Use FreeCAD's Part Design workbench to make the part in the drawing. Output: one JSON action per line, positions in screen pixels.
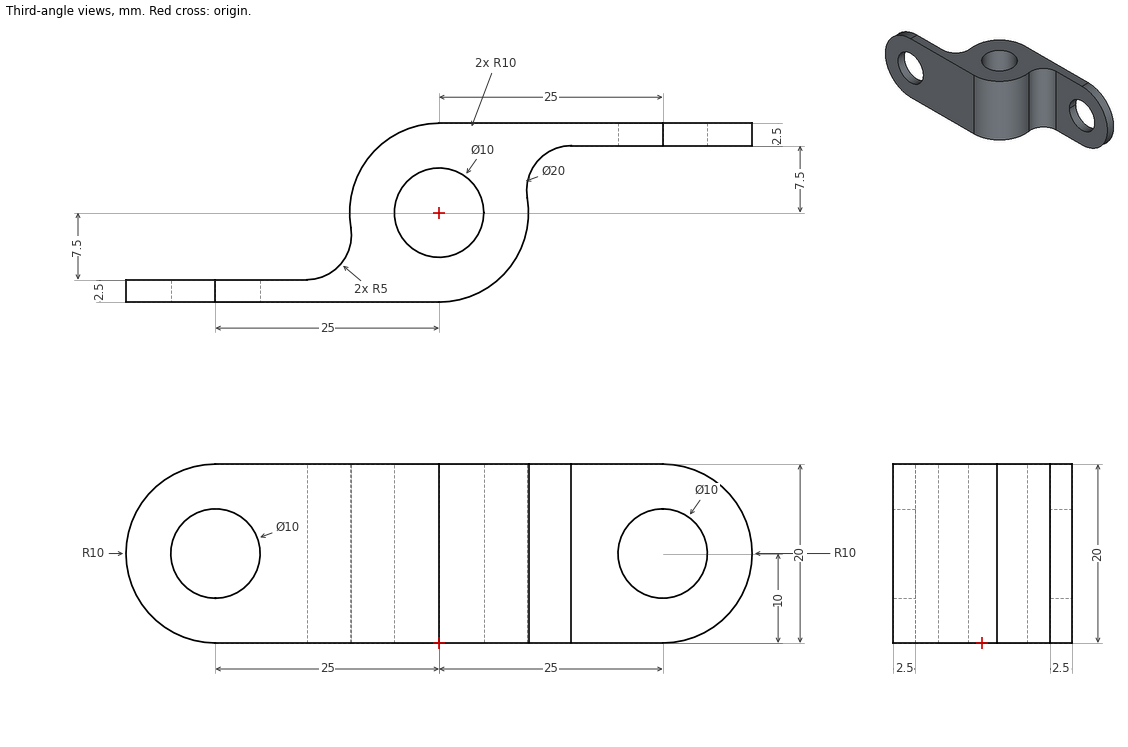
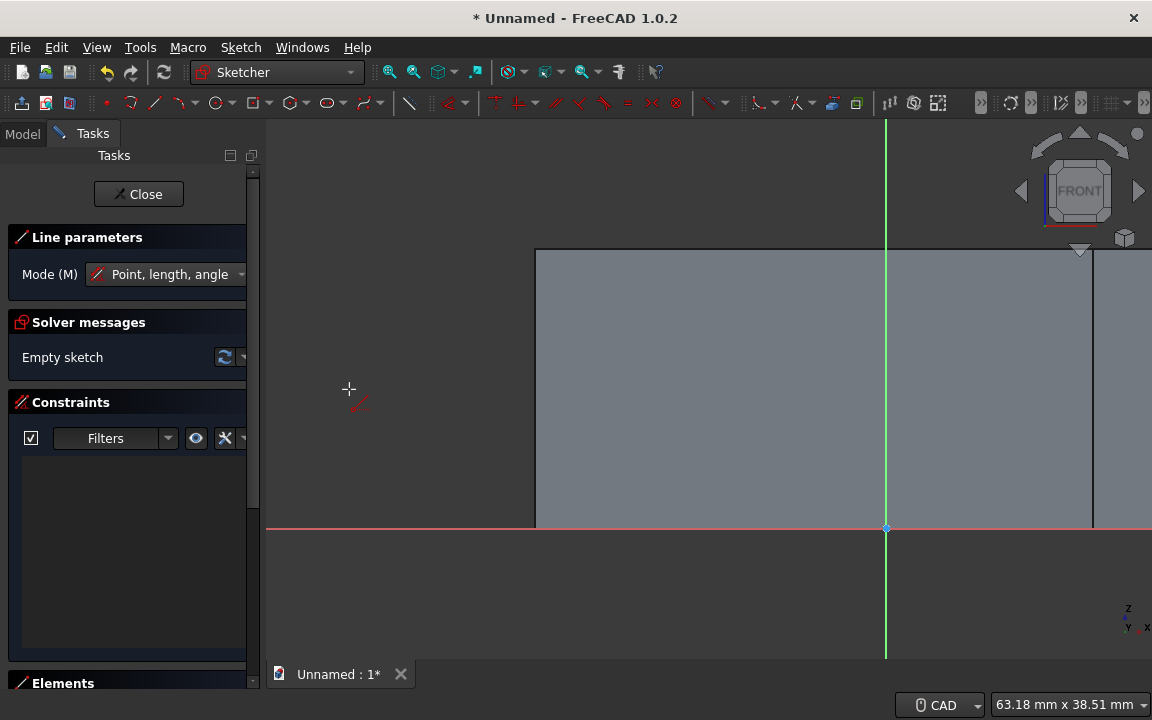
{"action": "left_click", "coordinate": [535, 529]}
{"action": "left_click", "coordinate": [535, 249]}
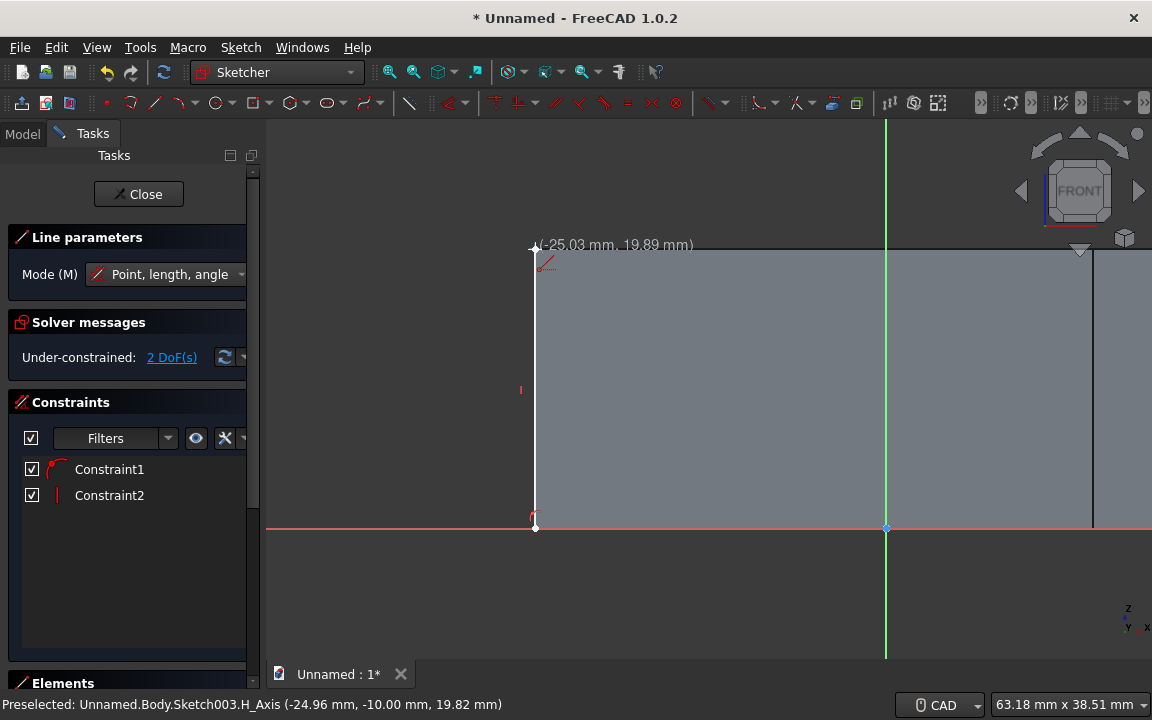
{"action": "left_click", "coordinate": [180, 104]}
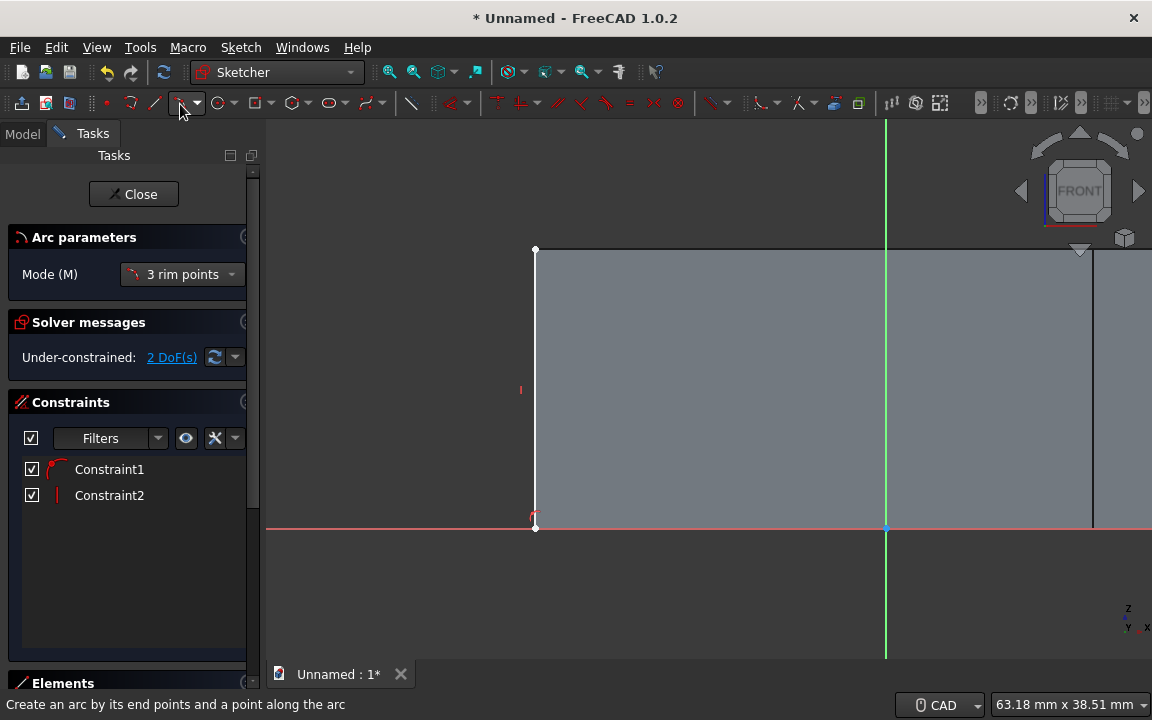
{"action": "left_click", "coordinate": [535, 250]}
{"action": "left_click", "coordinate": [535, 529]}
{"action": "left_click", "coordinate": [395, 389]}
{"action": "key", "text": "Escape"}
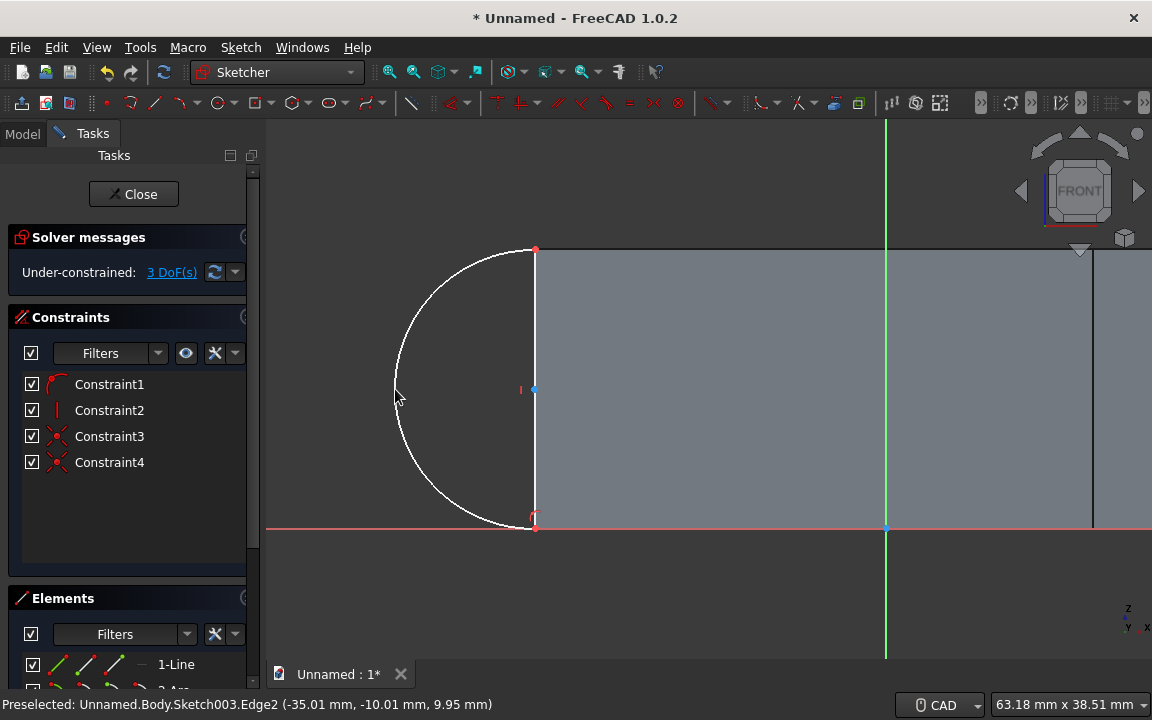
{"action": "key", "text": "d"}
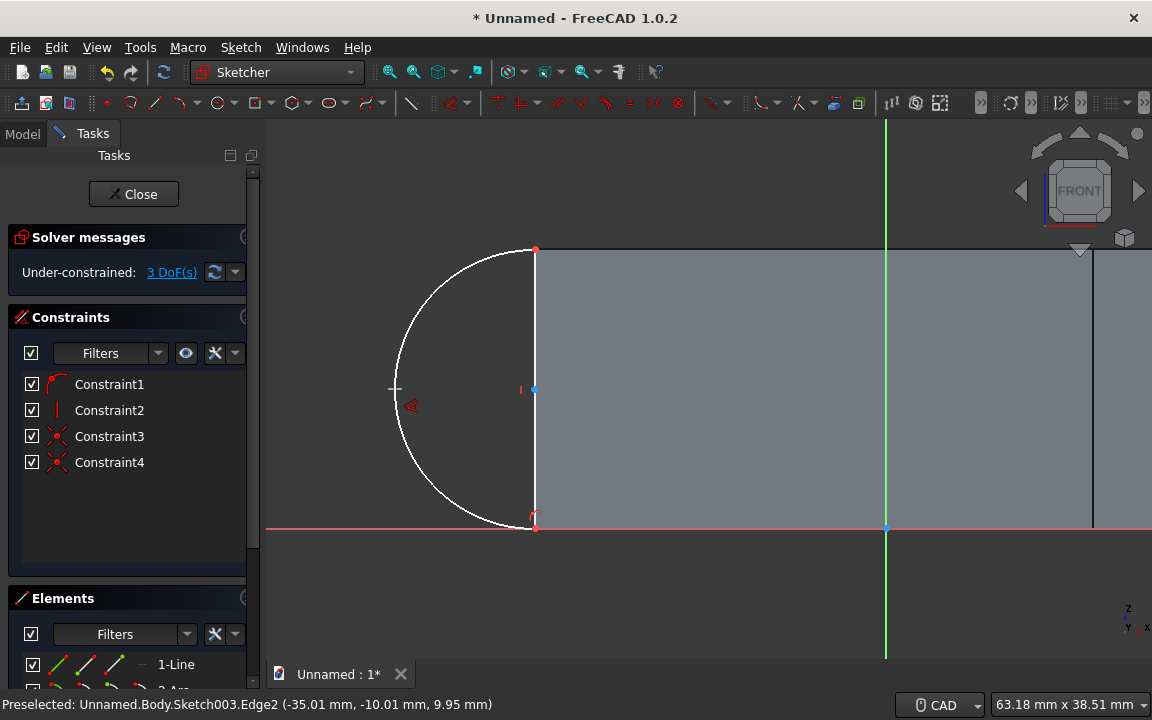
{"action": "left_click", "coordinate": [422, 307]}
{"action": "left_click", "coordinate": [396, 288]}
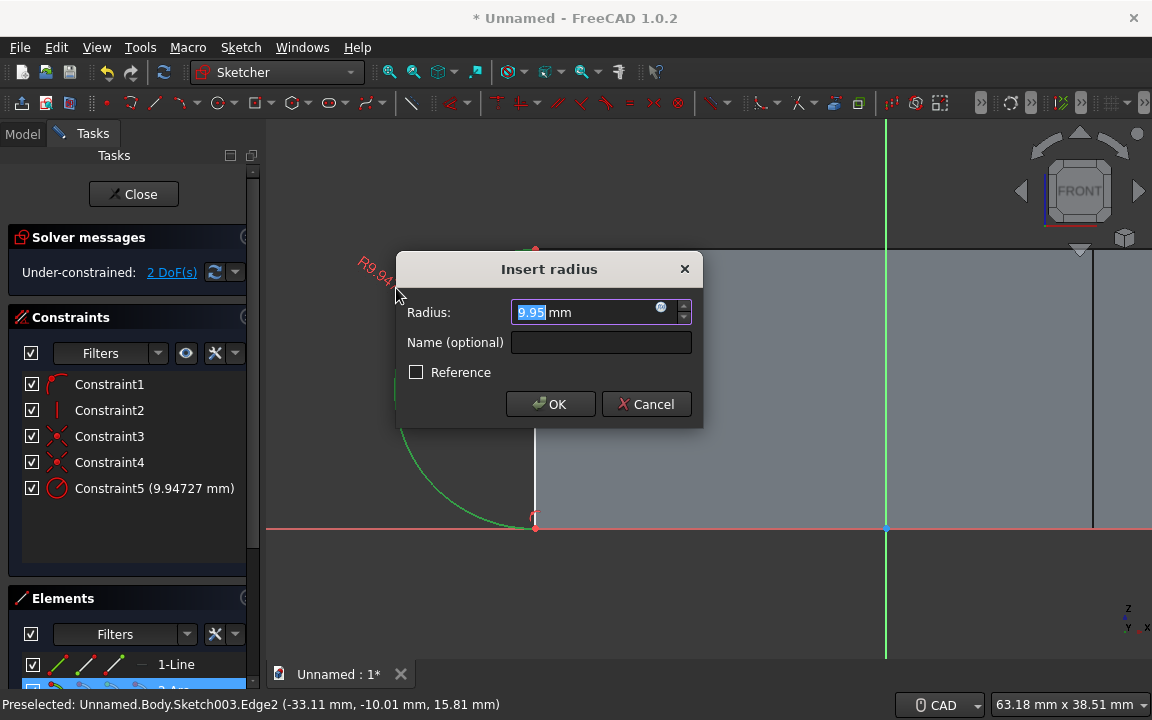
{"action": "type", "text": "10"}
{"action": "key", "text": "Return"}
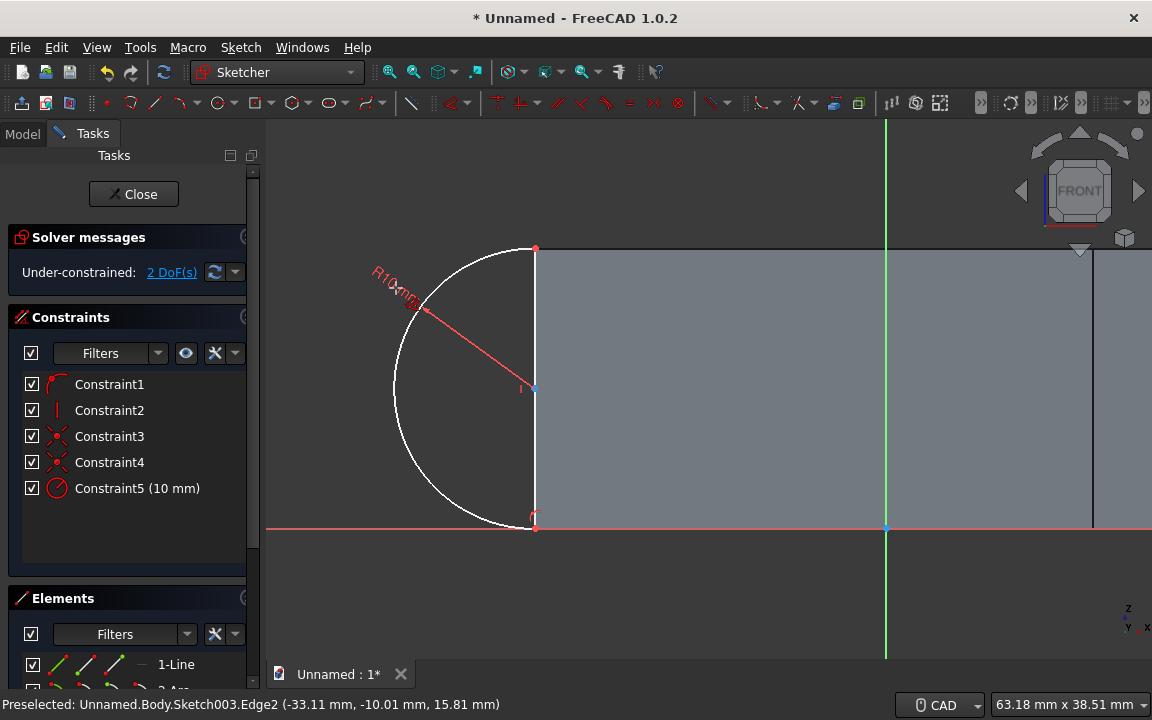
{"action": "left_click", "coordinate": [535, 529]}
{"action": "left_click", "coordinate": [711, 563]}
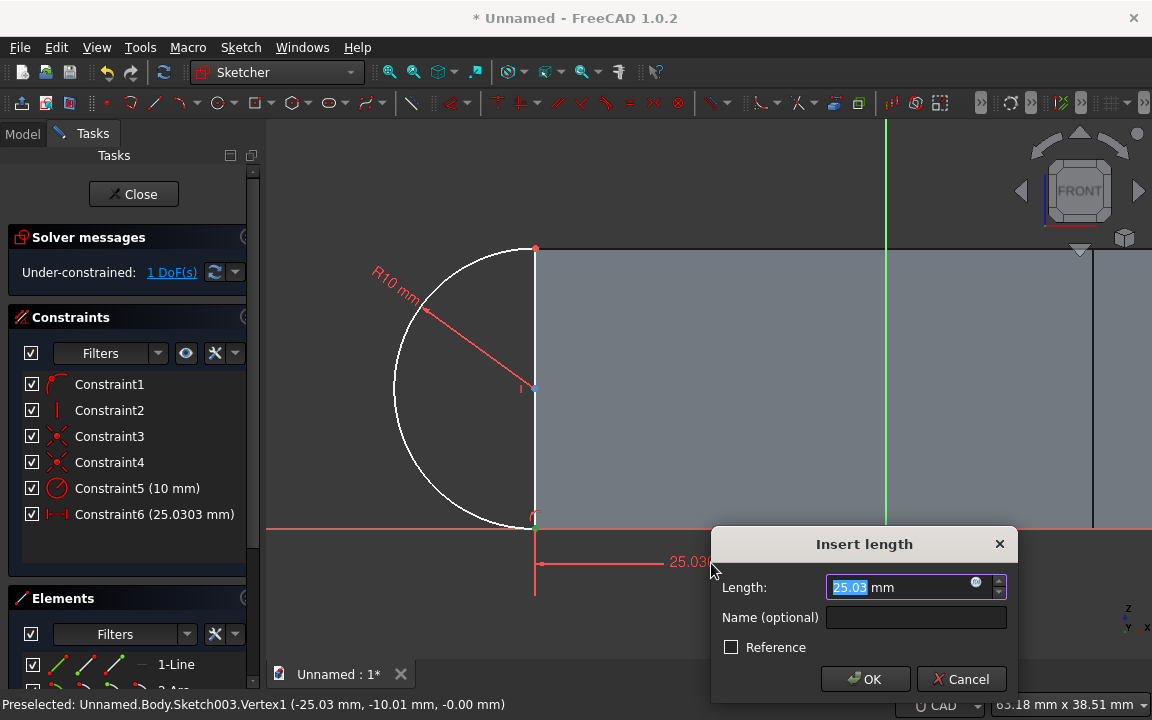
{"action": "type", "text": "25"}
{"action": "key", "text": "Return"}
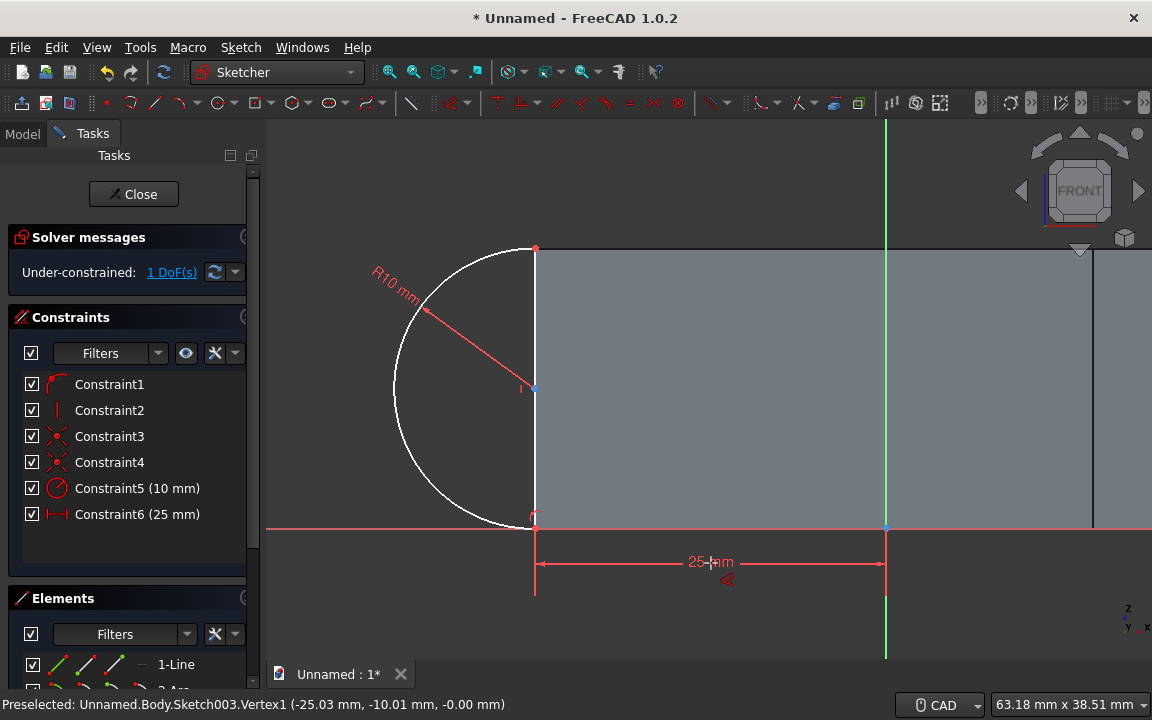
{"action": "left_click", "coordinate": [534, 389]}
{"action": "left_click", "coordinate": [629, 563]}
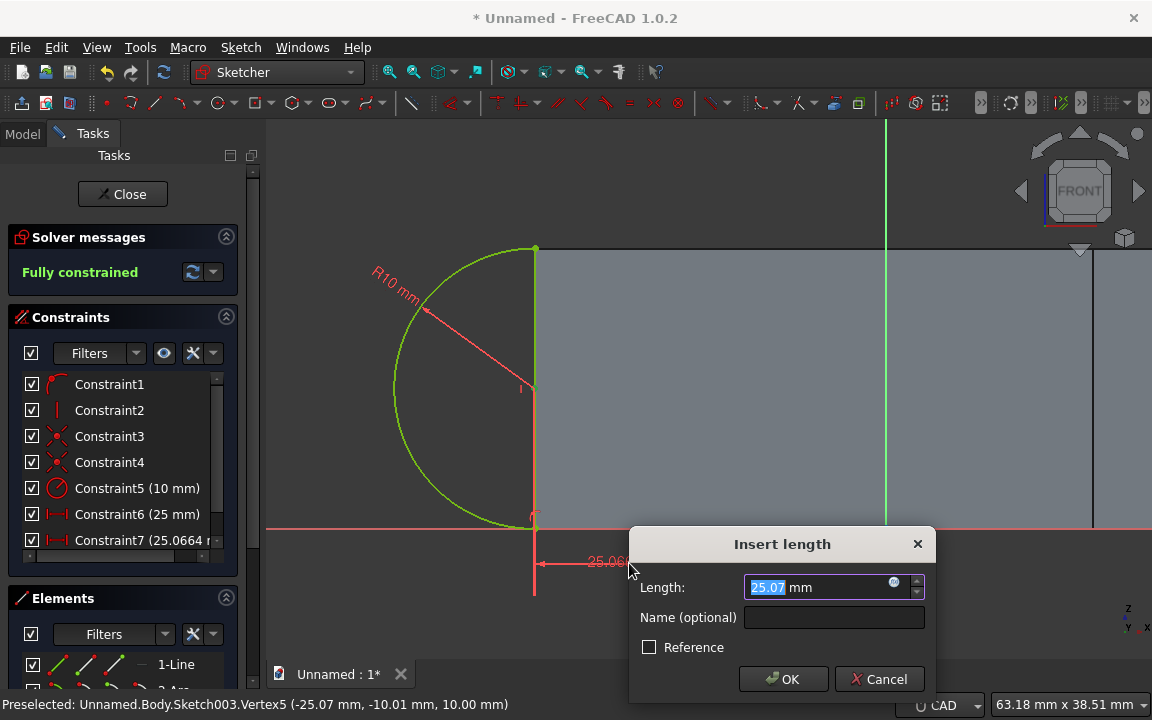
{"action": "type", "text": "25"}
{"action": "key", "text": "Return"}
{"action": "key", "text": "Escape"}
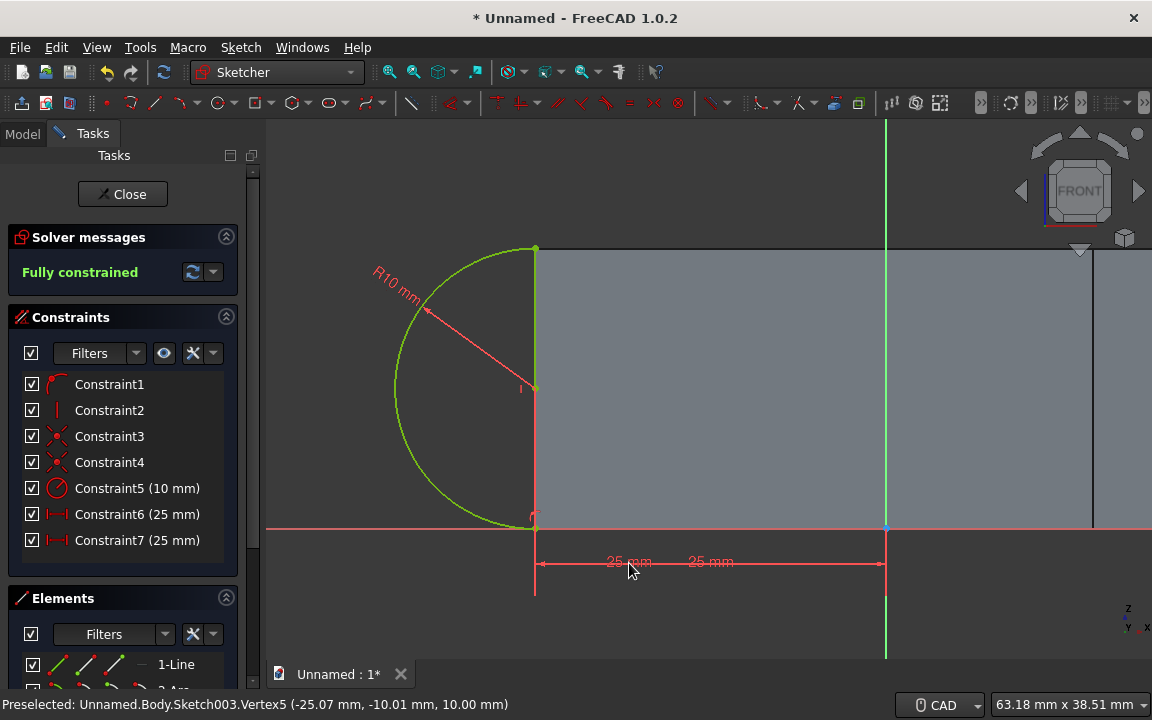
{"action": "left_click", "coordinate": [123, 194]}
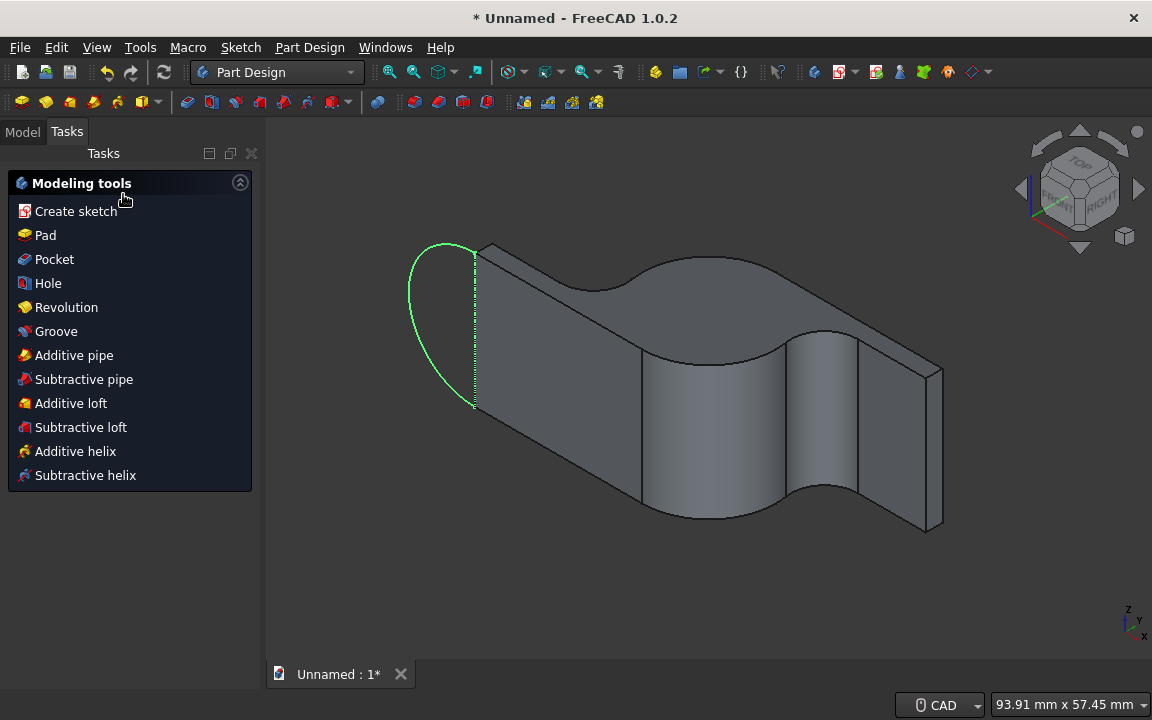
{"action": "left_click", "coordinate": [22, 102]}